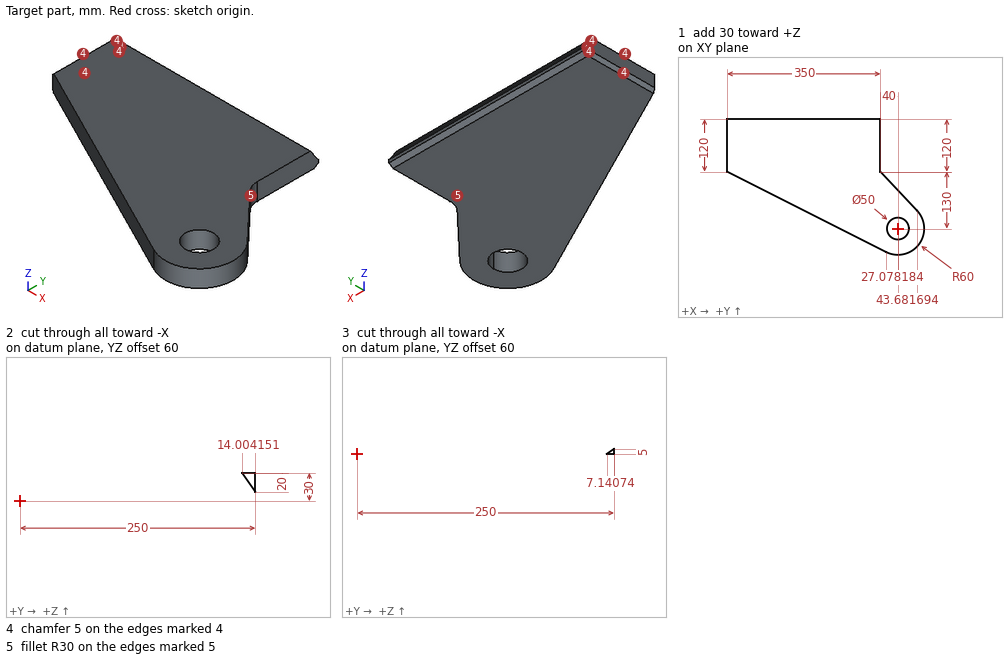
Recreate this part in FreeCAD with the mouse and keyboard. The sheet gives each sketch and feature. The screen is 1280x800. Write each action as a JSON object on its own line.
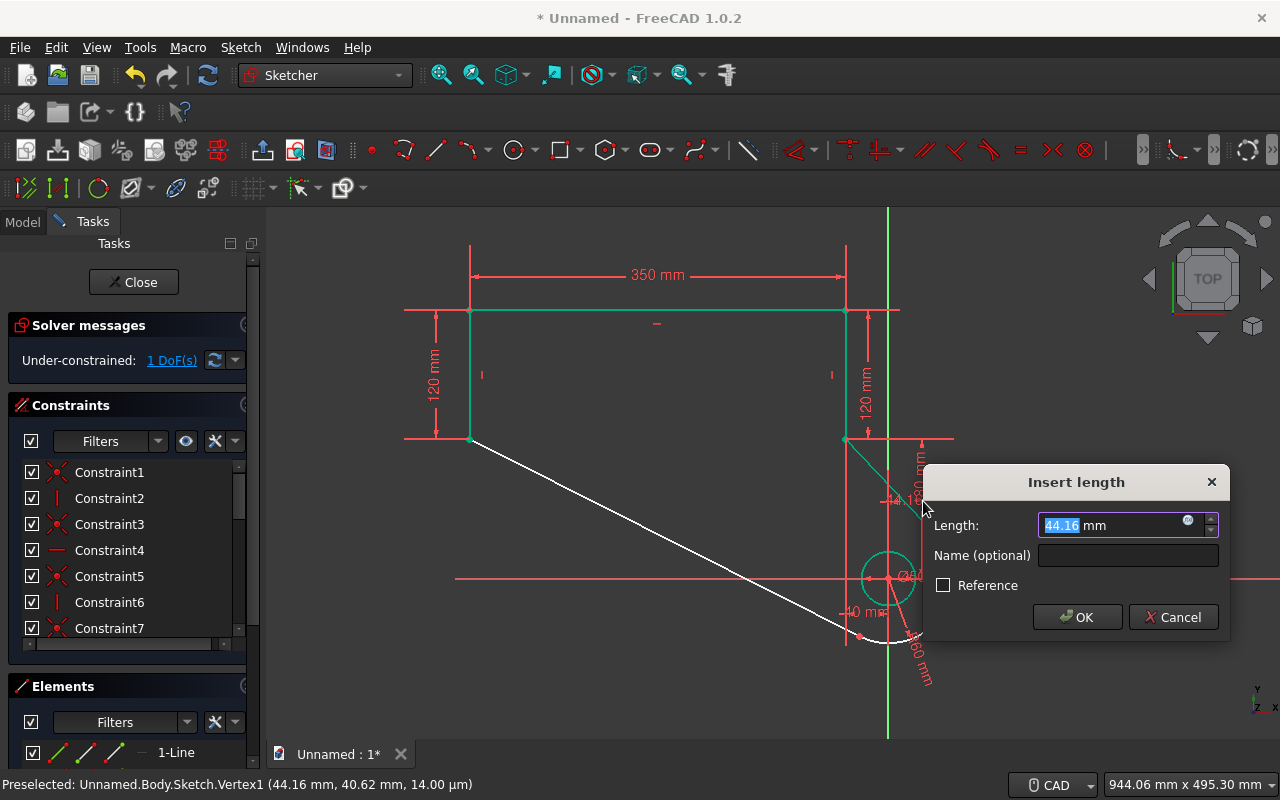
{"action": "type", "text": "43.681694"}
{"action": "key", "text": "Return"}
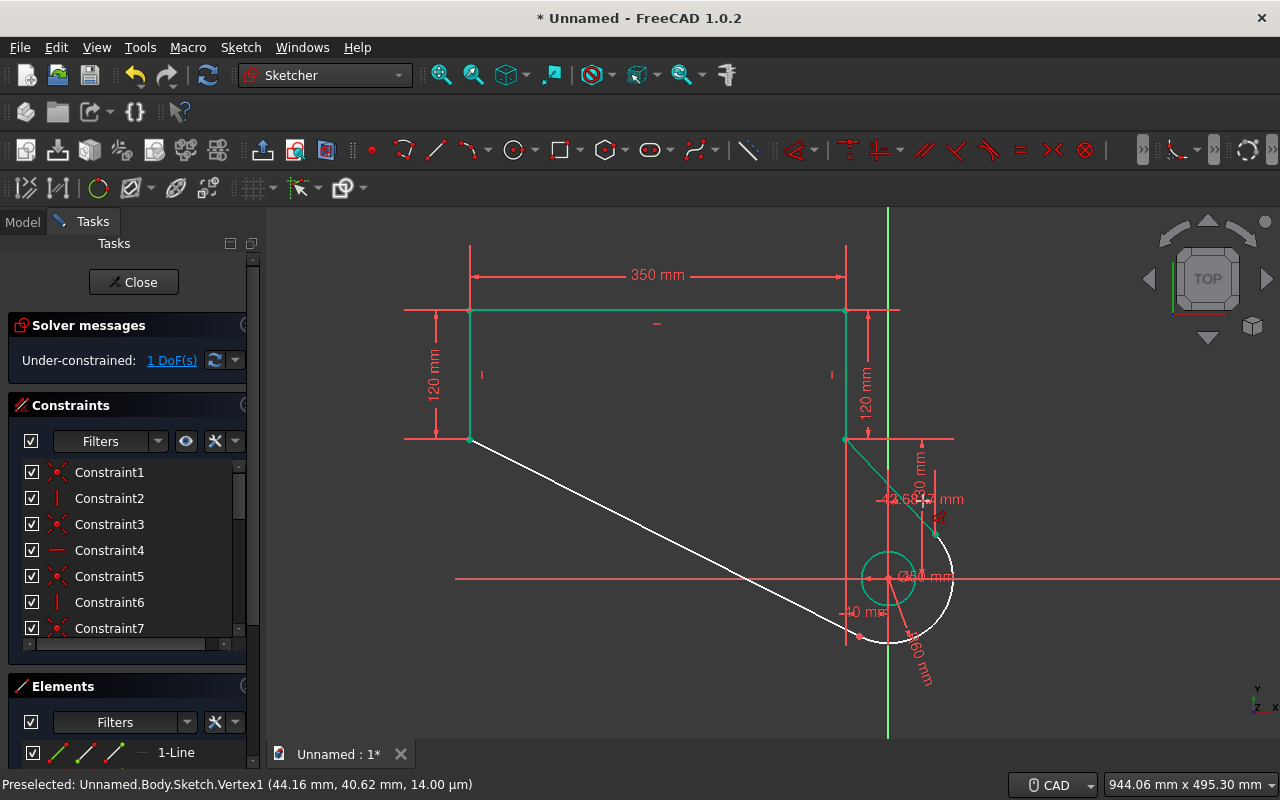
{"action": "scroll", "coordinate": [859, 636], "scroll_direction": "up", "scroll_amount": 2}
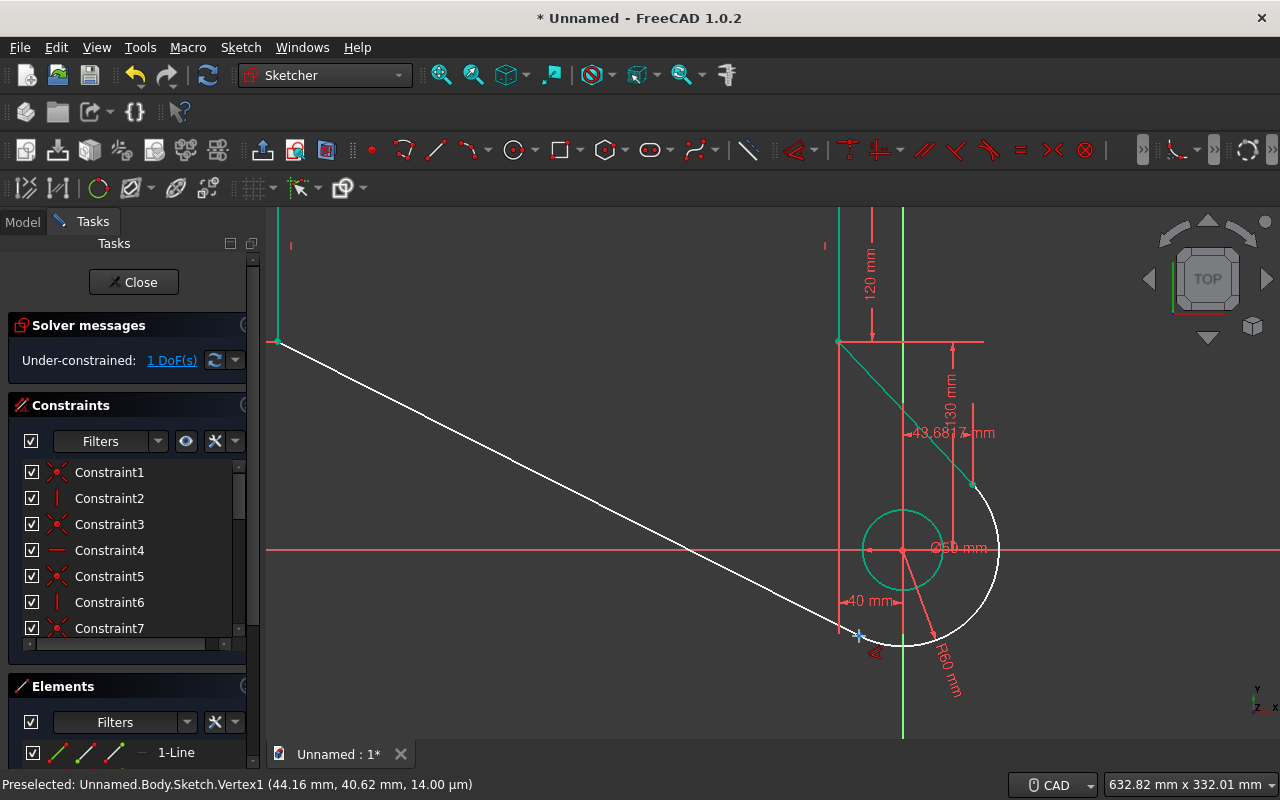
{"action": "left_click", "coordinate": [859, 636]}
{"action": "left_click", "coordinate": [871, 670]}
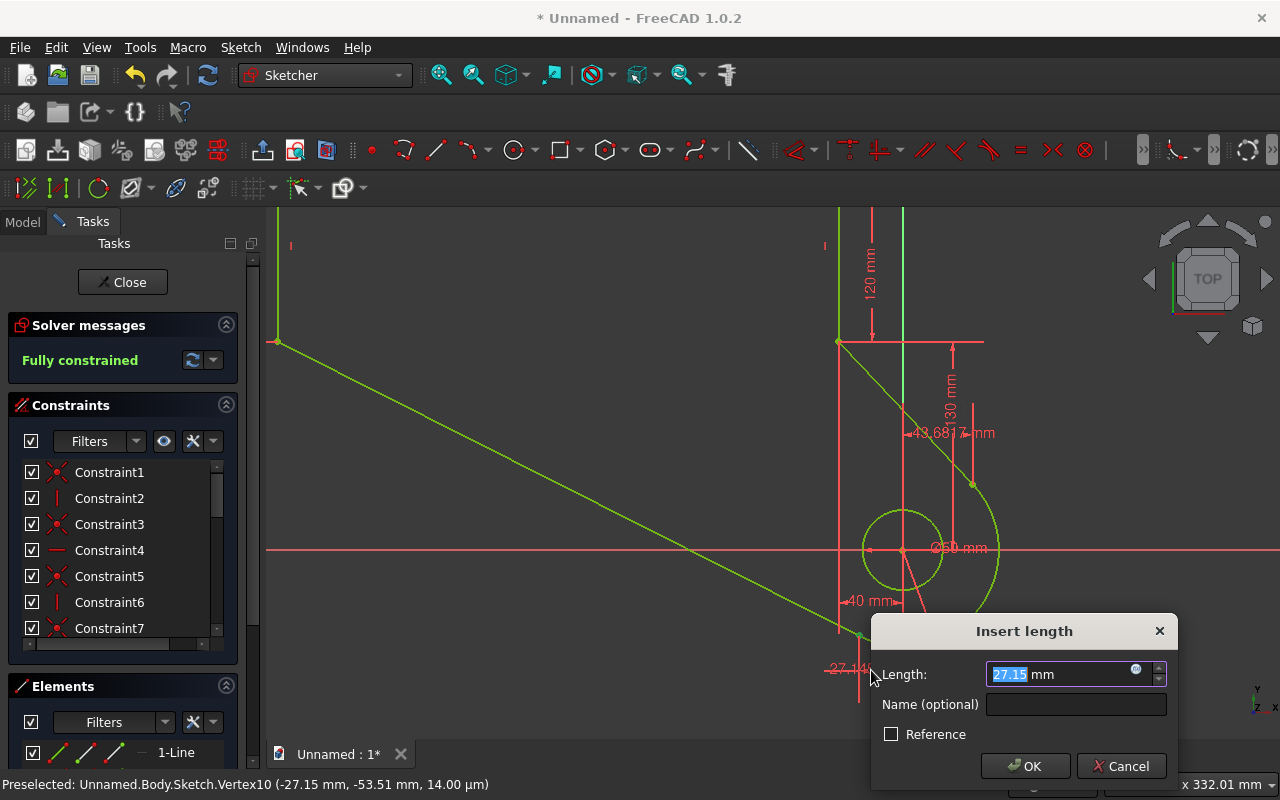
{"action": "type", "text": "27.078184"}
{"action": "key", "text": "Return"}
{"action": "key", "text": "Escape"}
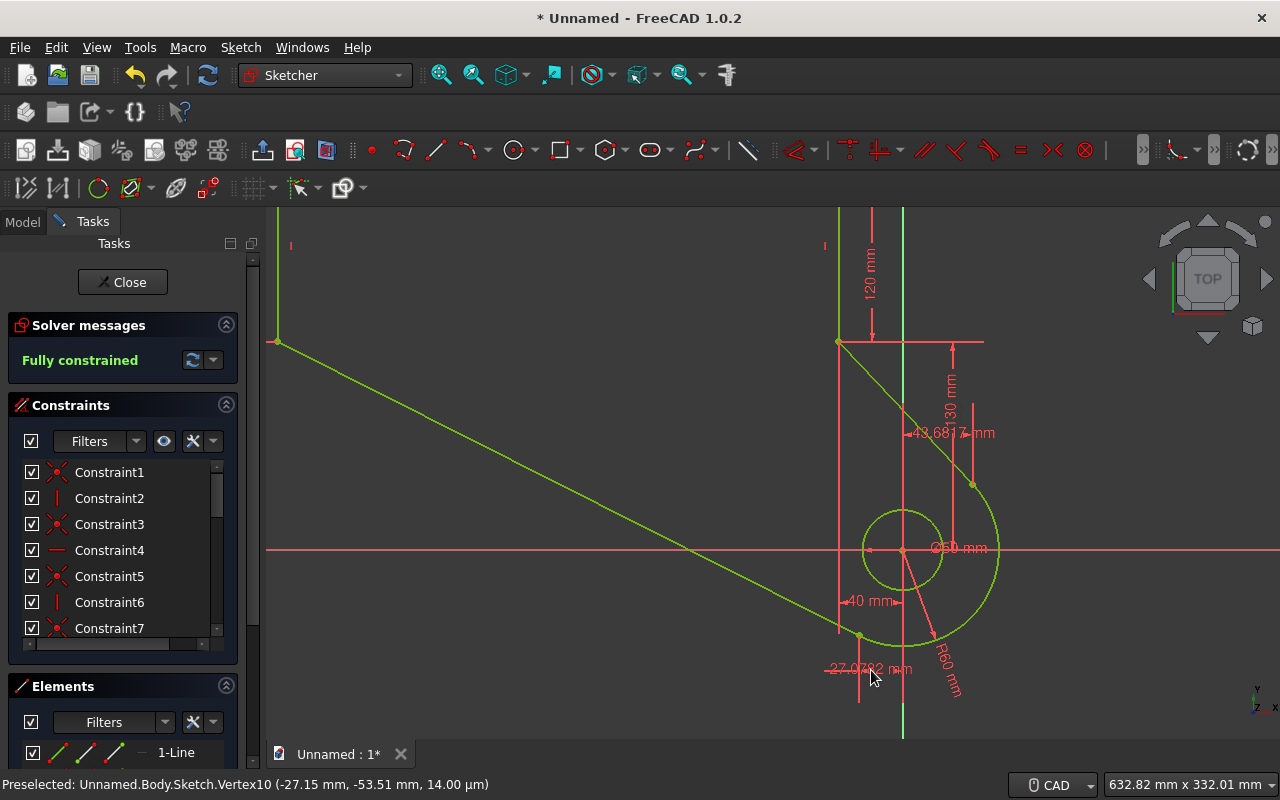
{"action": "left_click", "coordinate": [123, 282]}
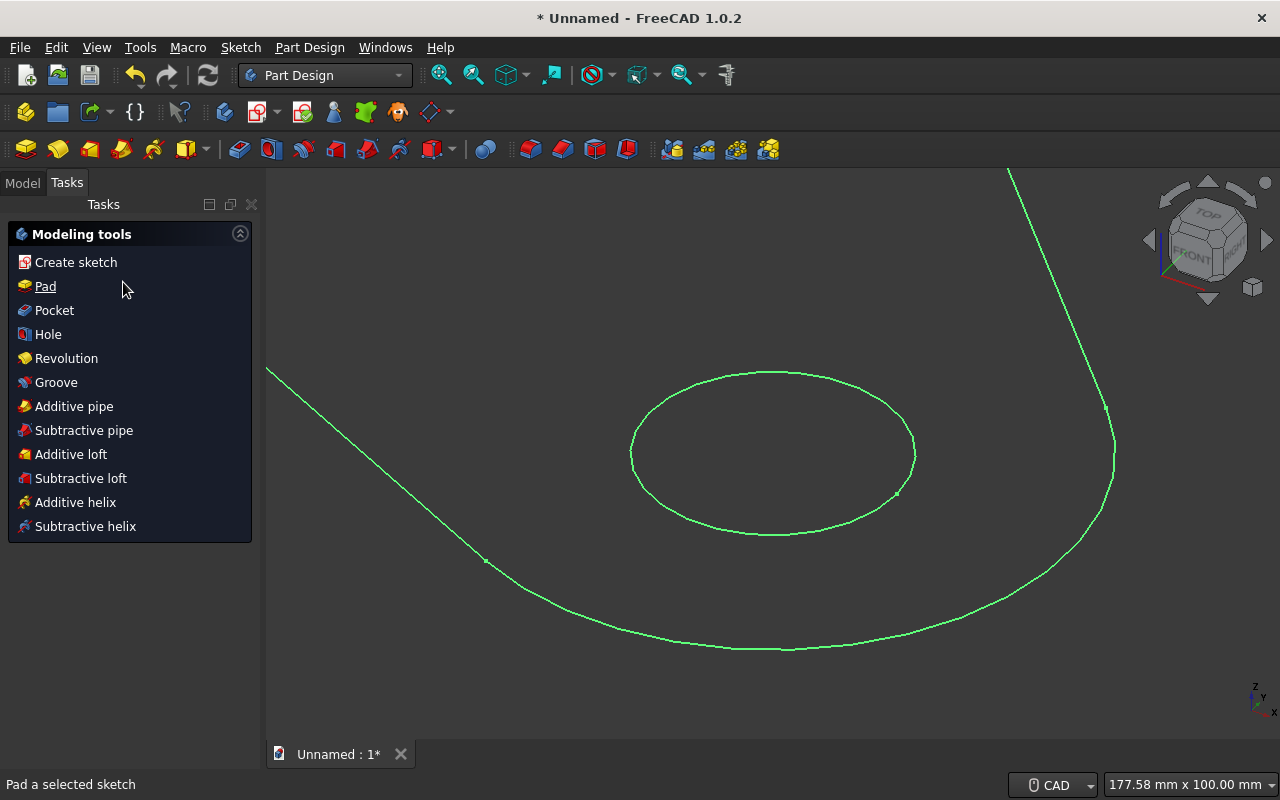
{"action": "left_click", "coordinate": [26, 150]}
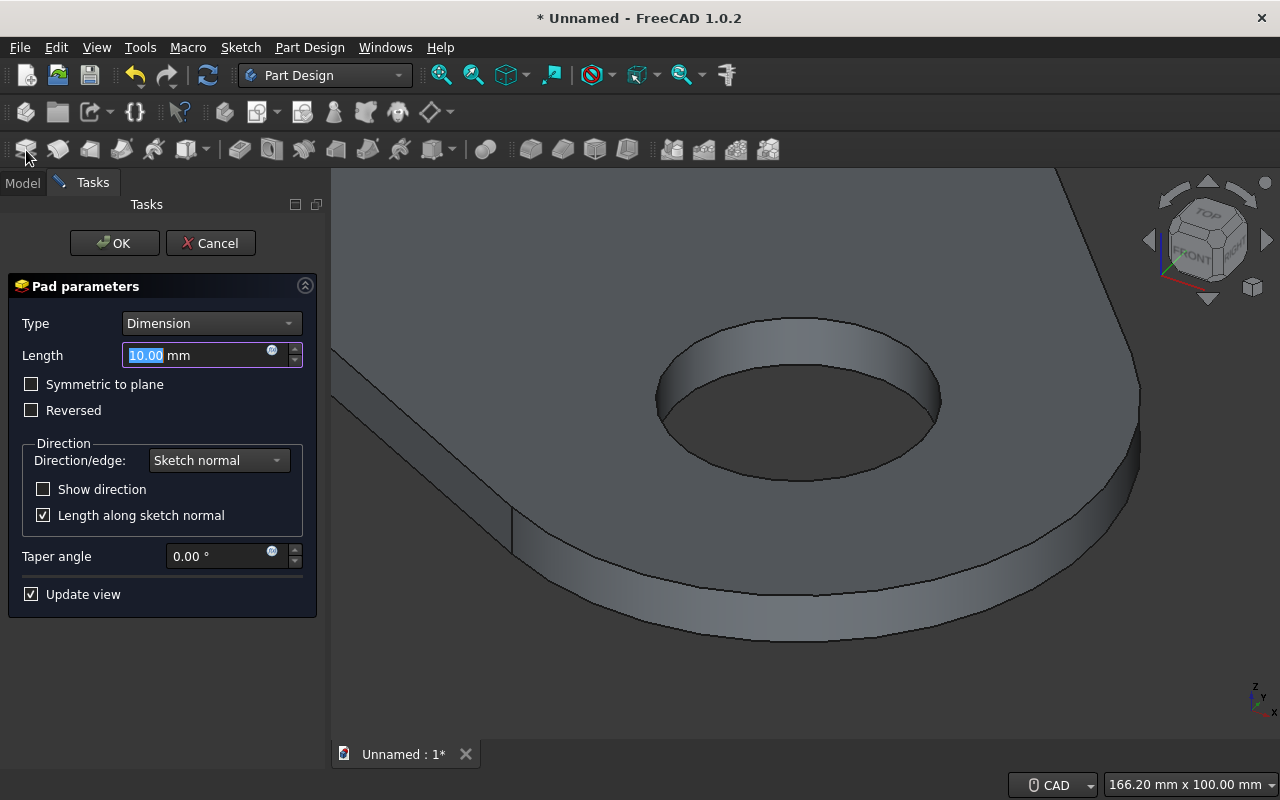
{"action": "type", "text": "30"}
{"action": "key", "text": "Tab"}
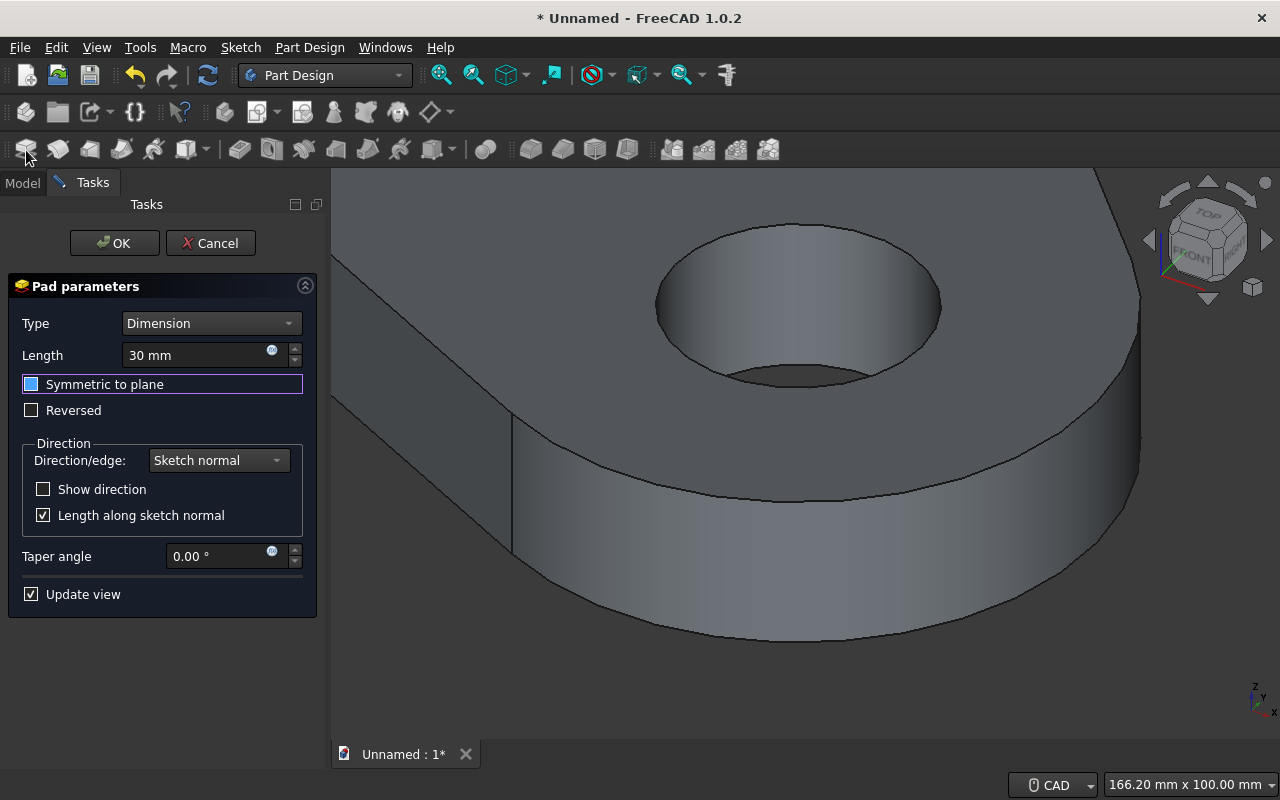
{"action": "left_click", "coordinate": [115, 243]}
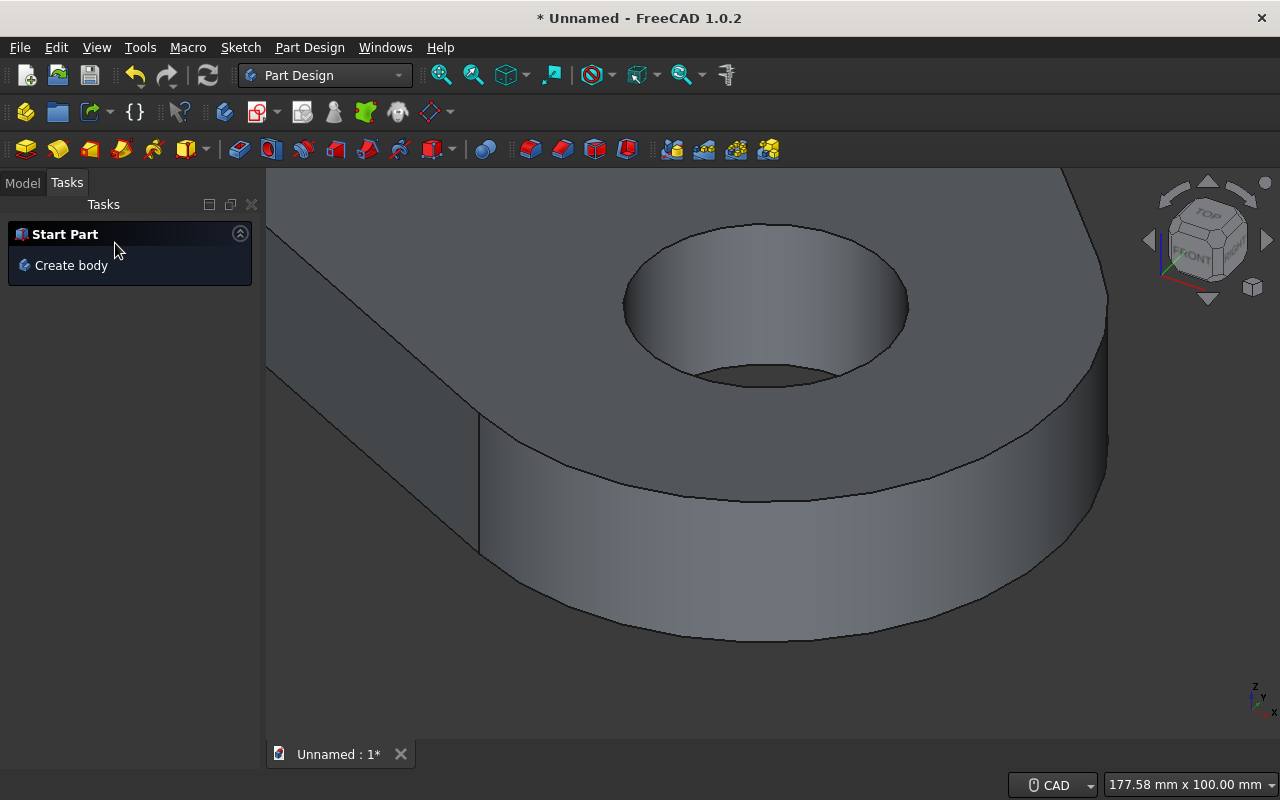
{"action": "key", "text": "v f"}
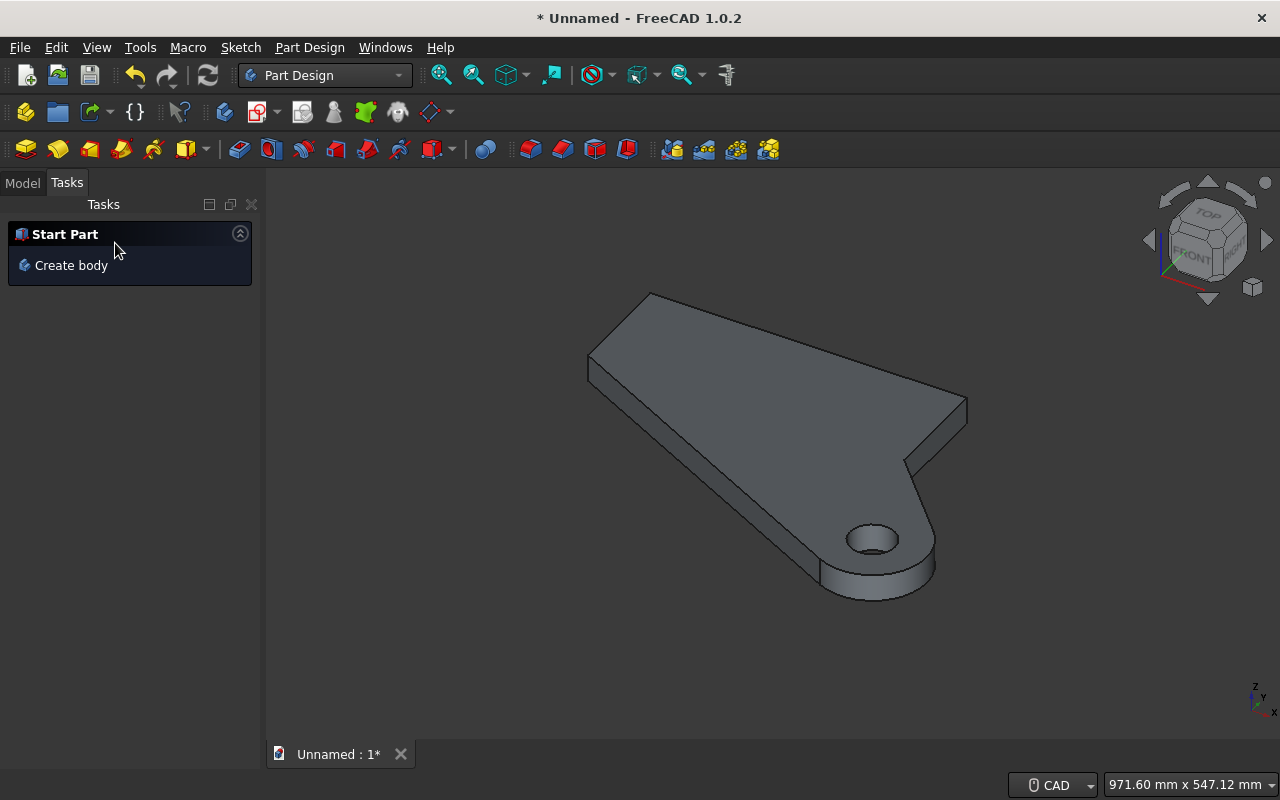
{"action": "left_click", "coordinate": [23, 182]}